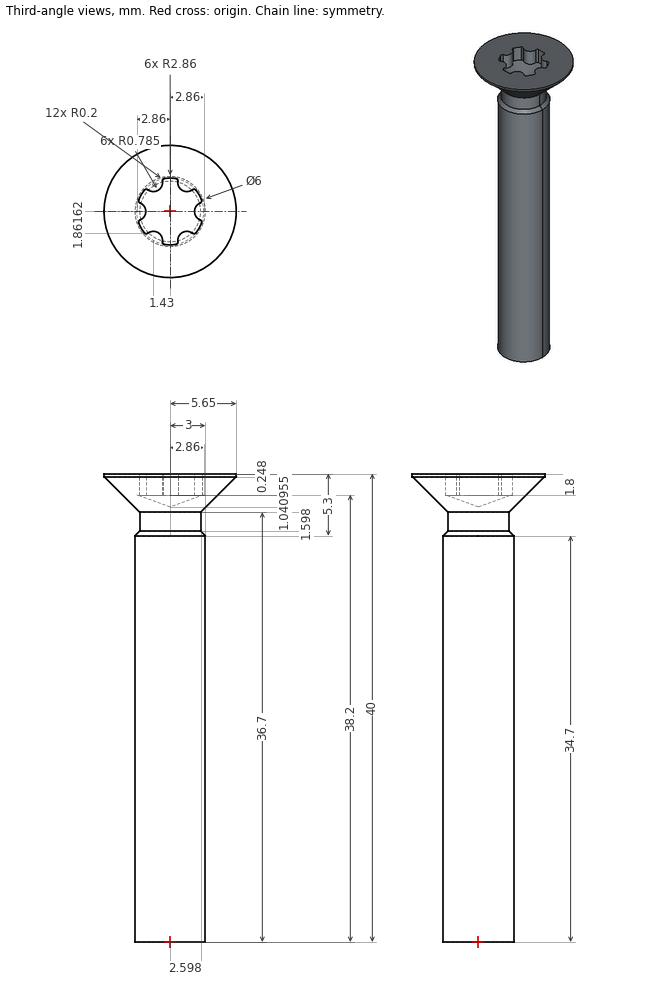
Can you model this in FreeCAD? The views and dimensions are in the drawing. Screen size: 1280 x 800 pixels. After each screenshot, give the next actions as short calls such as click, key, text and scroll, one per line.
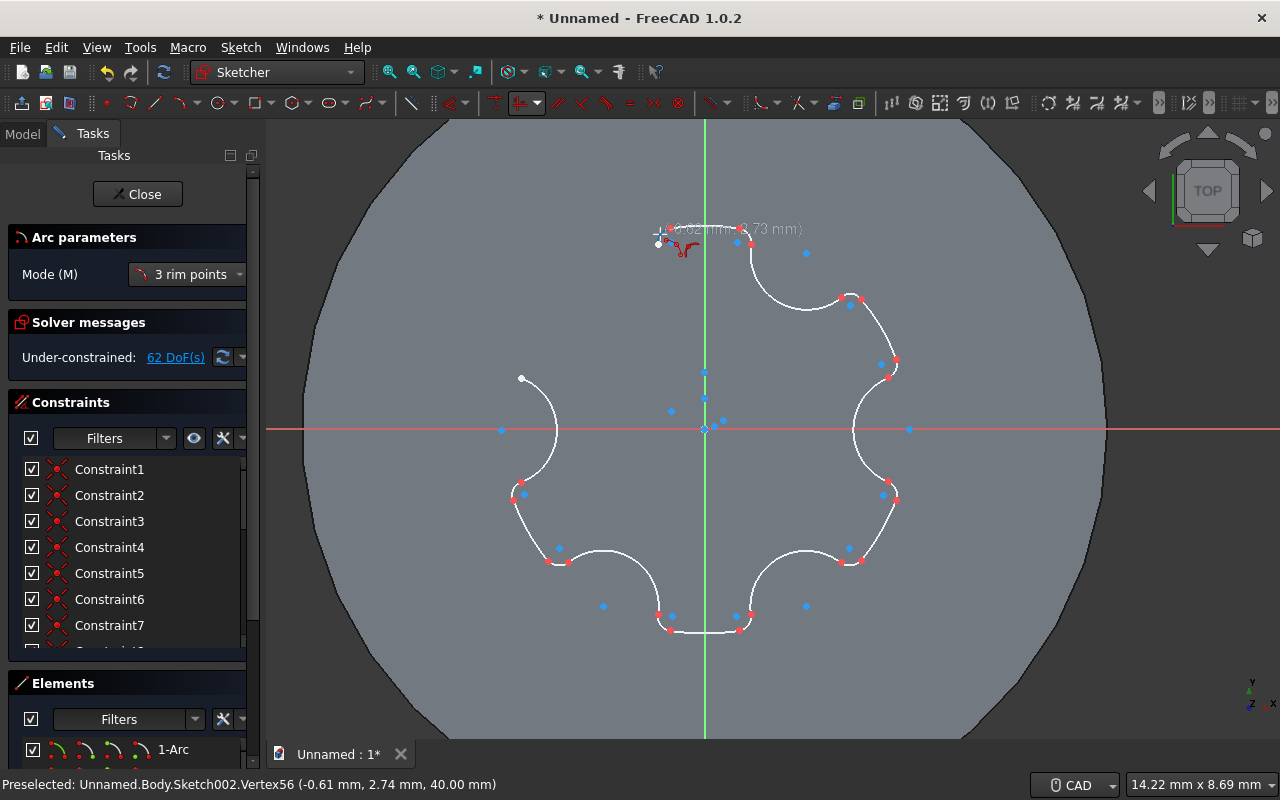
click(658, 245)
click(568, 297)
click(631, 301)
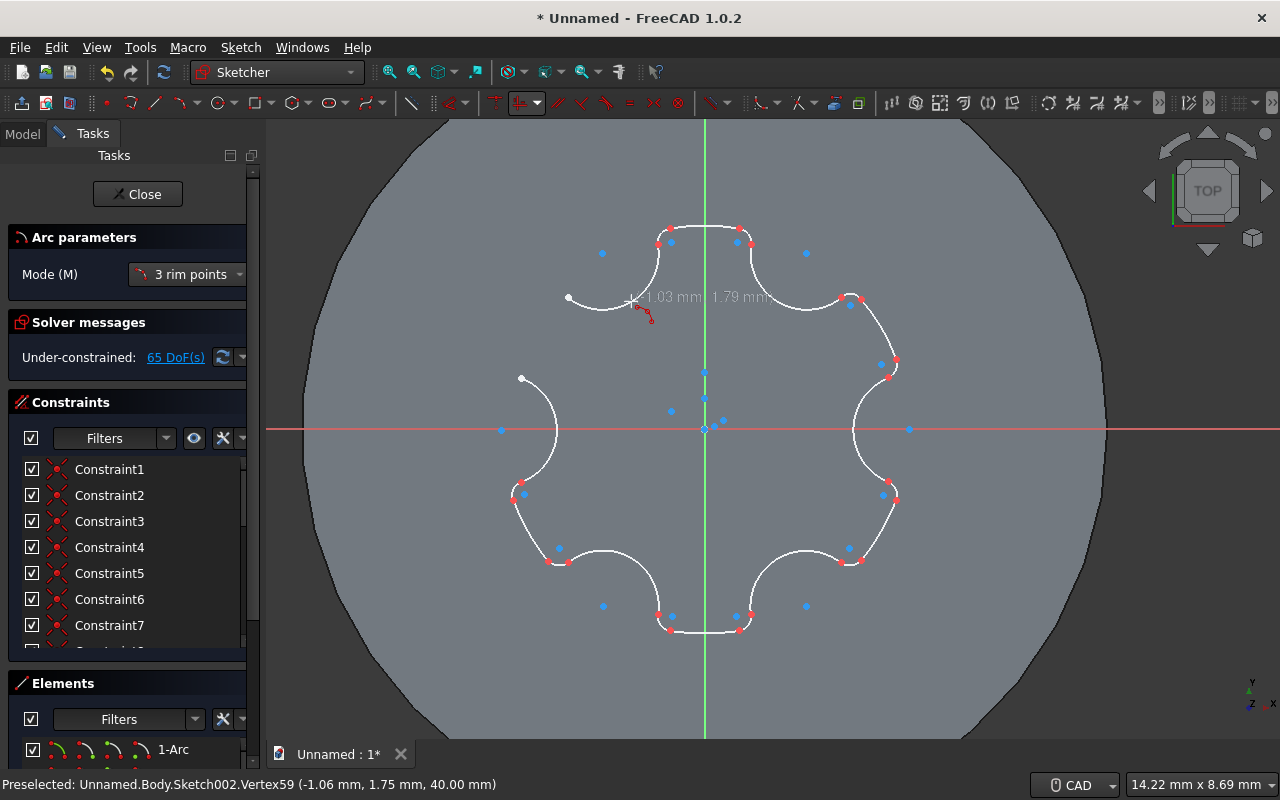
click(568, 298)
click(548, 299)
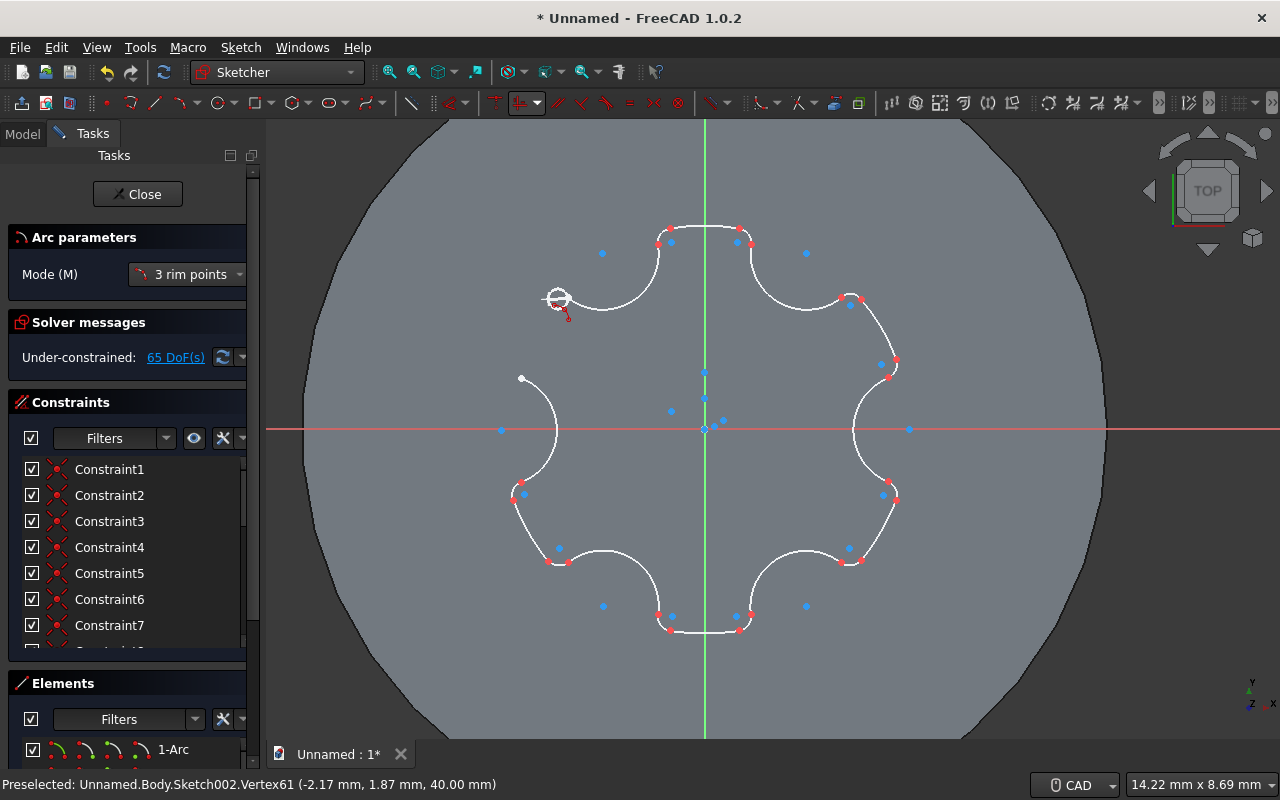
scroll(557, 294, up, 7)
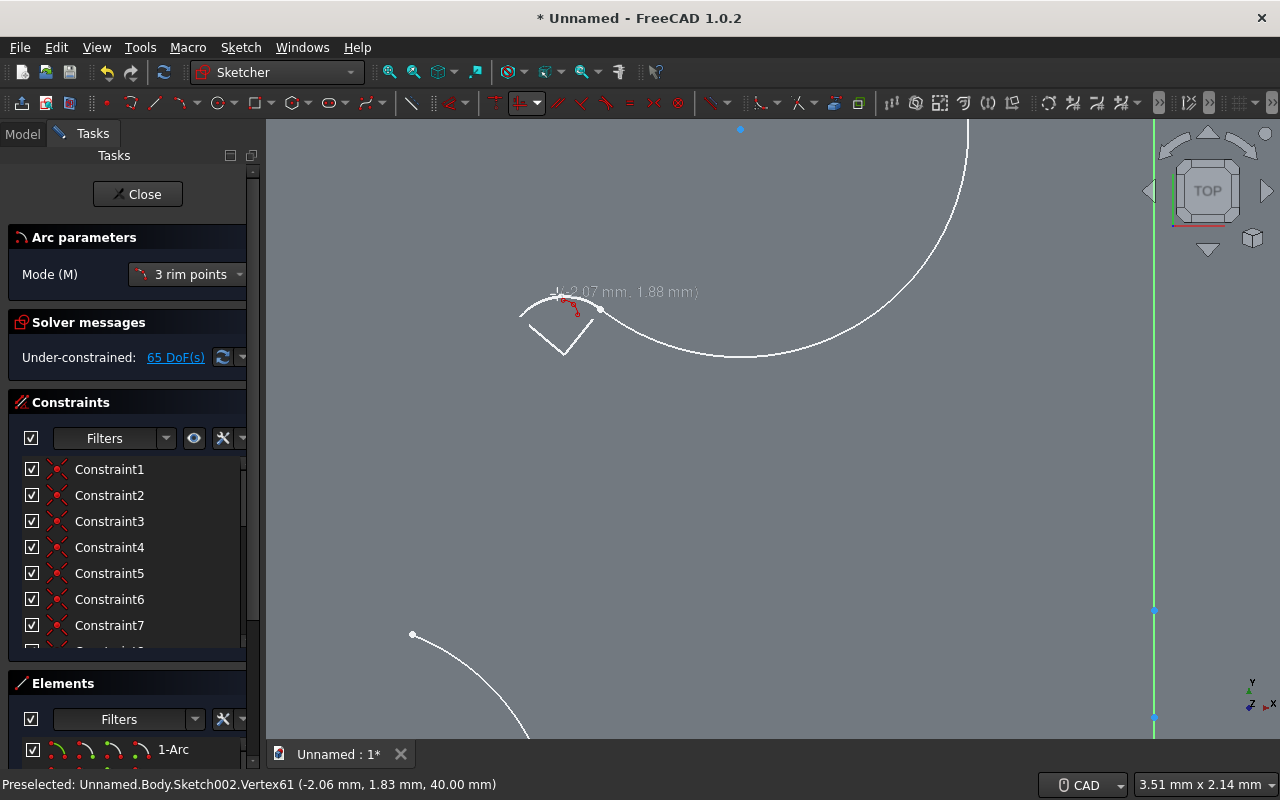
click(558, 291)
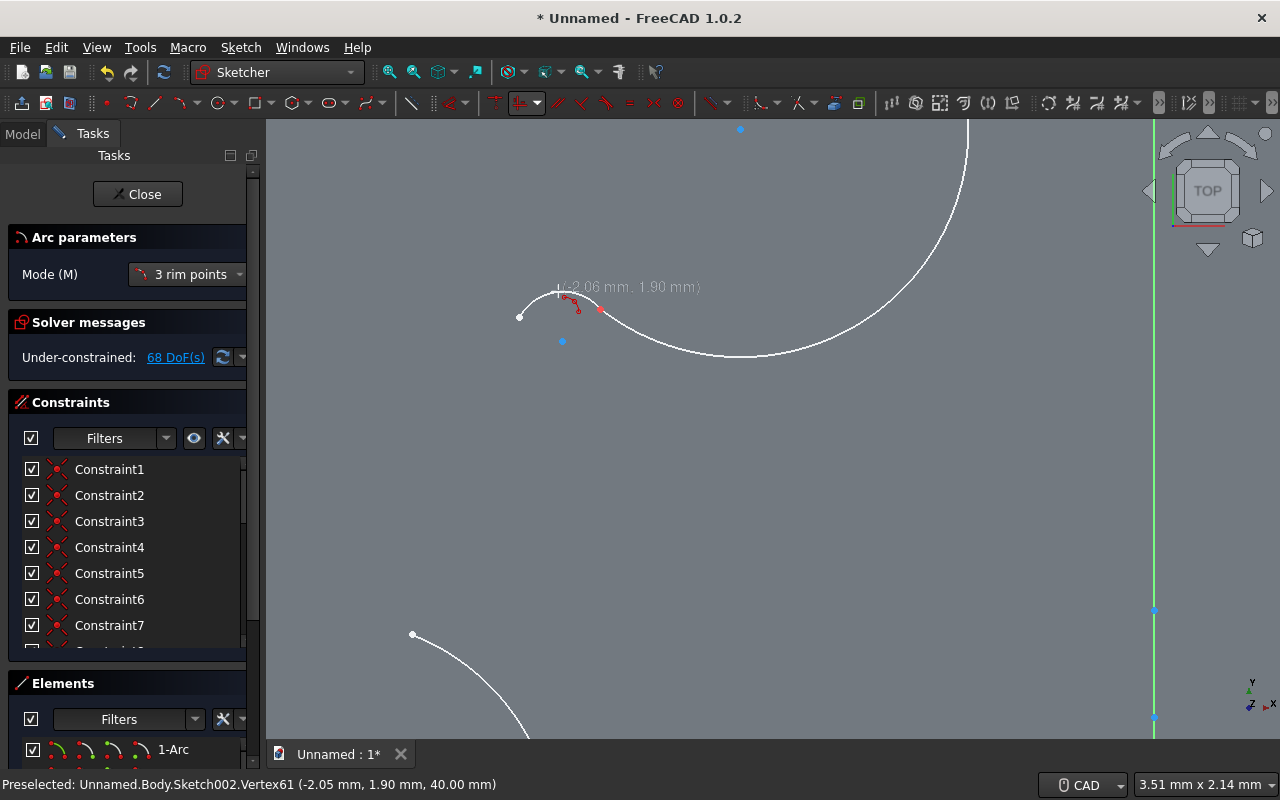
scroll(557, 294, down, 7)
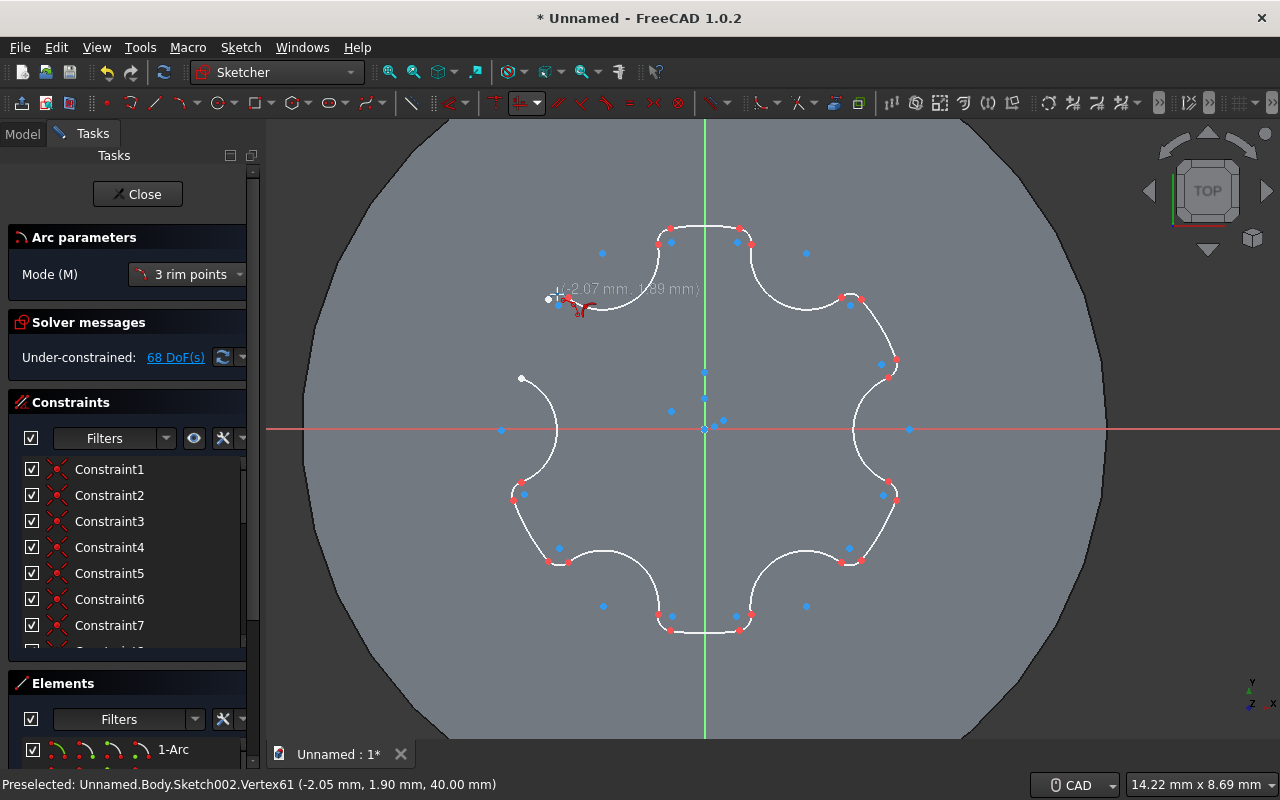
click(548, 300)
click(513, 359)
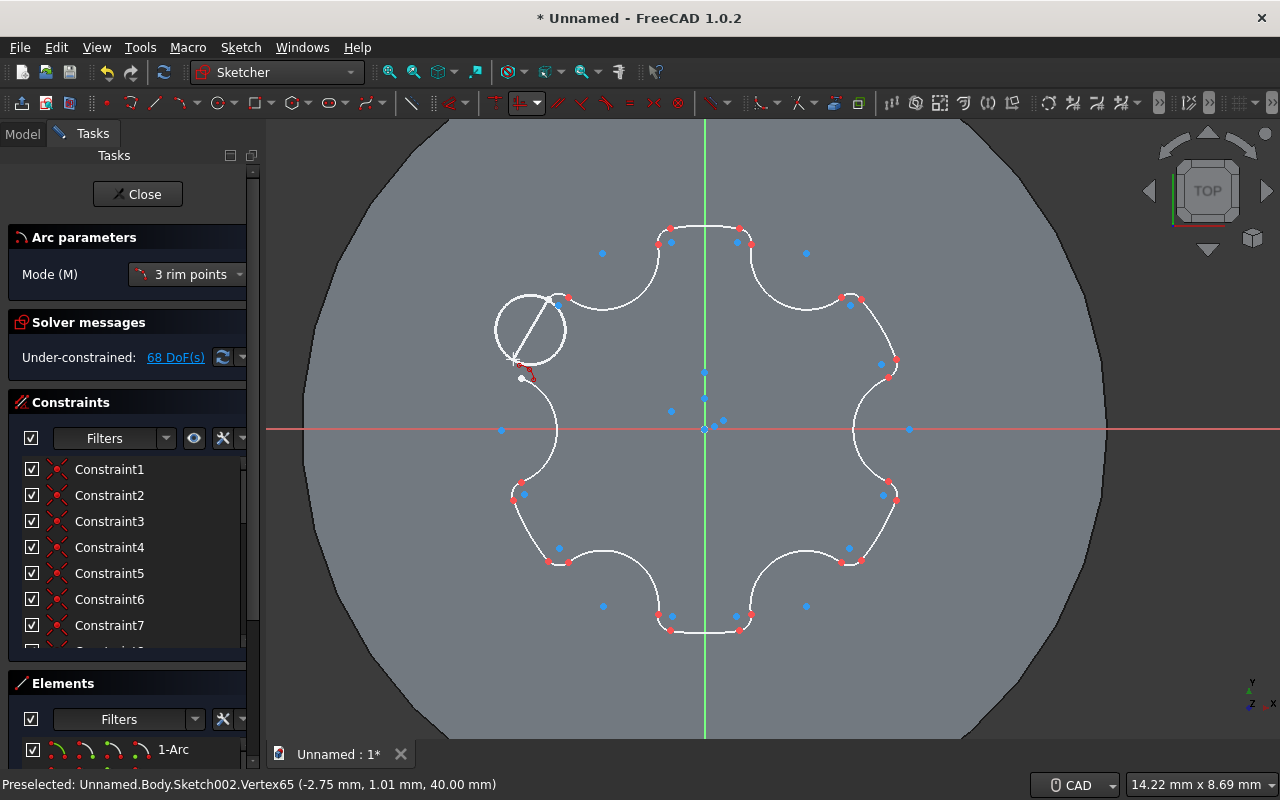
scroll(528, 327, up, 9)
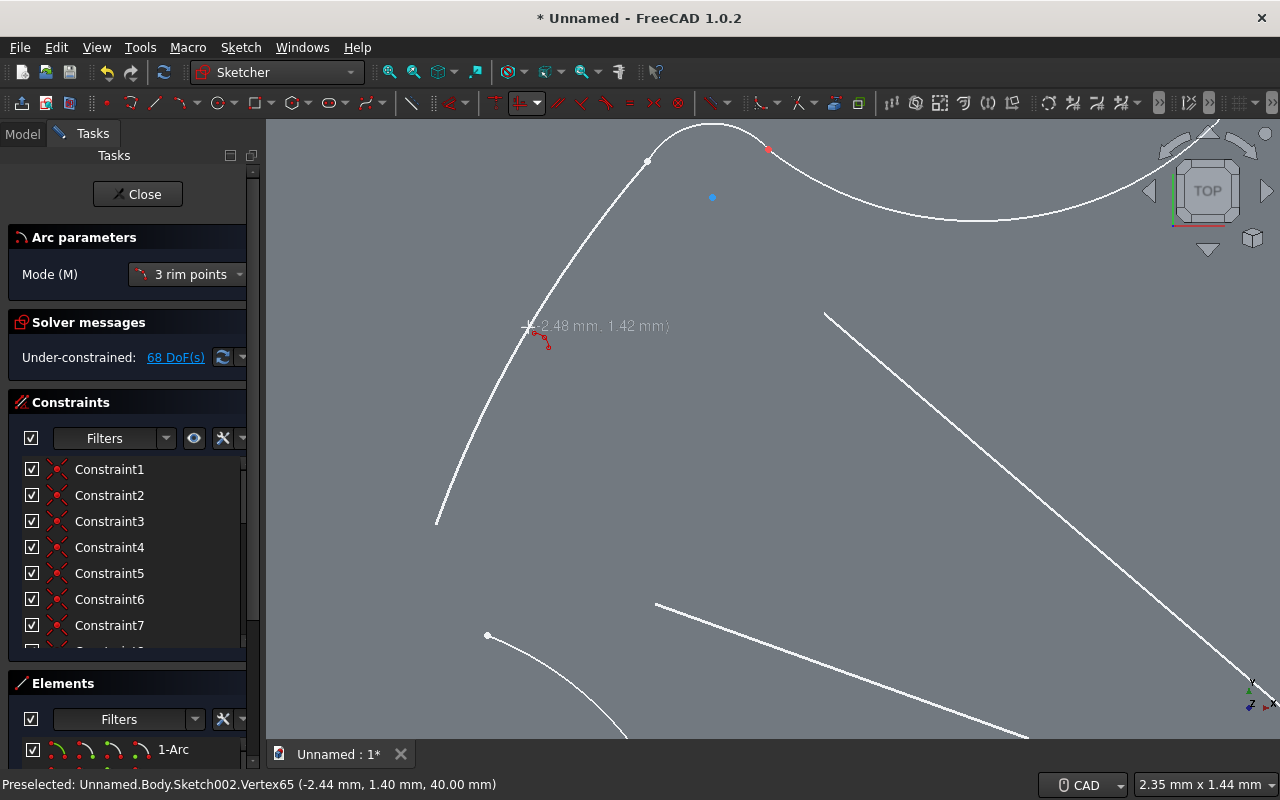
click(526, 327)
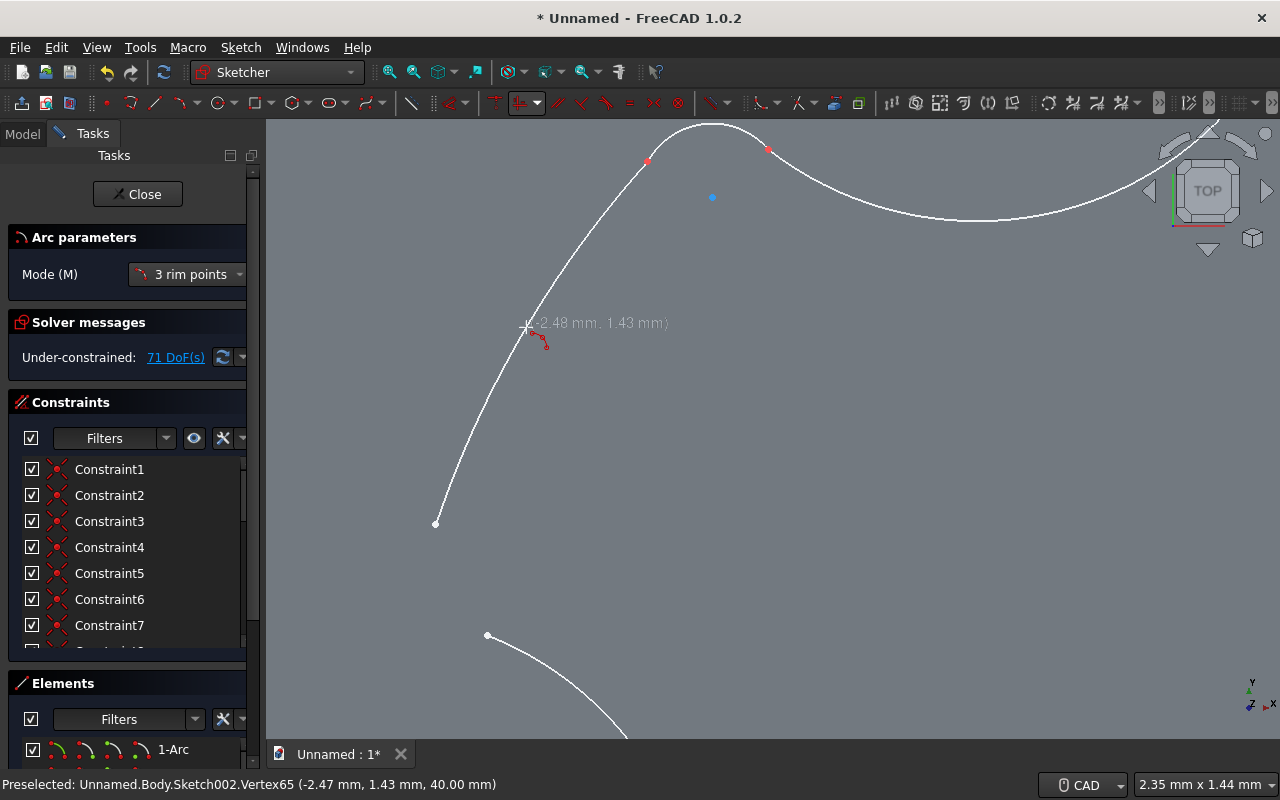
scroll(528, 327, down, 9)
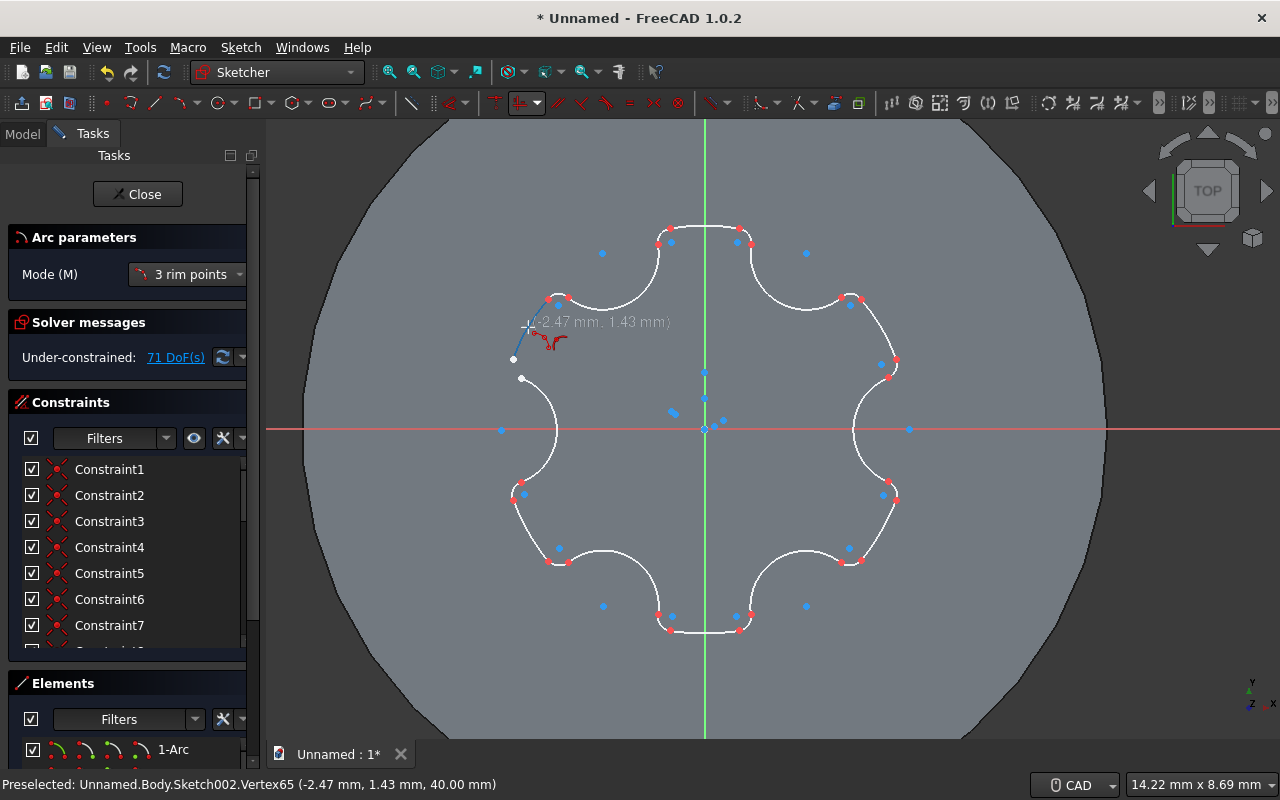
click(513, 360)
click(522, 378)